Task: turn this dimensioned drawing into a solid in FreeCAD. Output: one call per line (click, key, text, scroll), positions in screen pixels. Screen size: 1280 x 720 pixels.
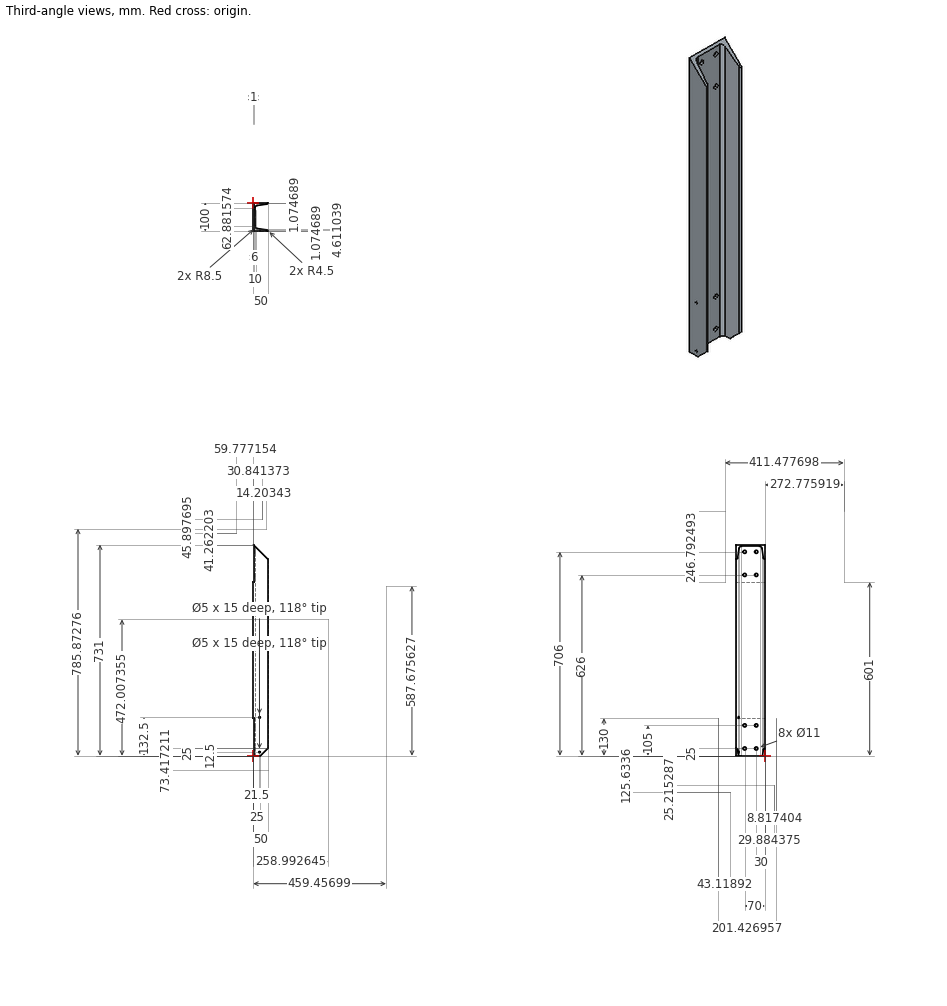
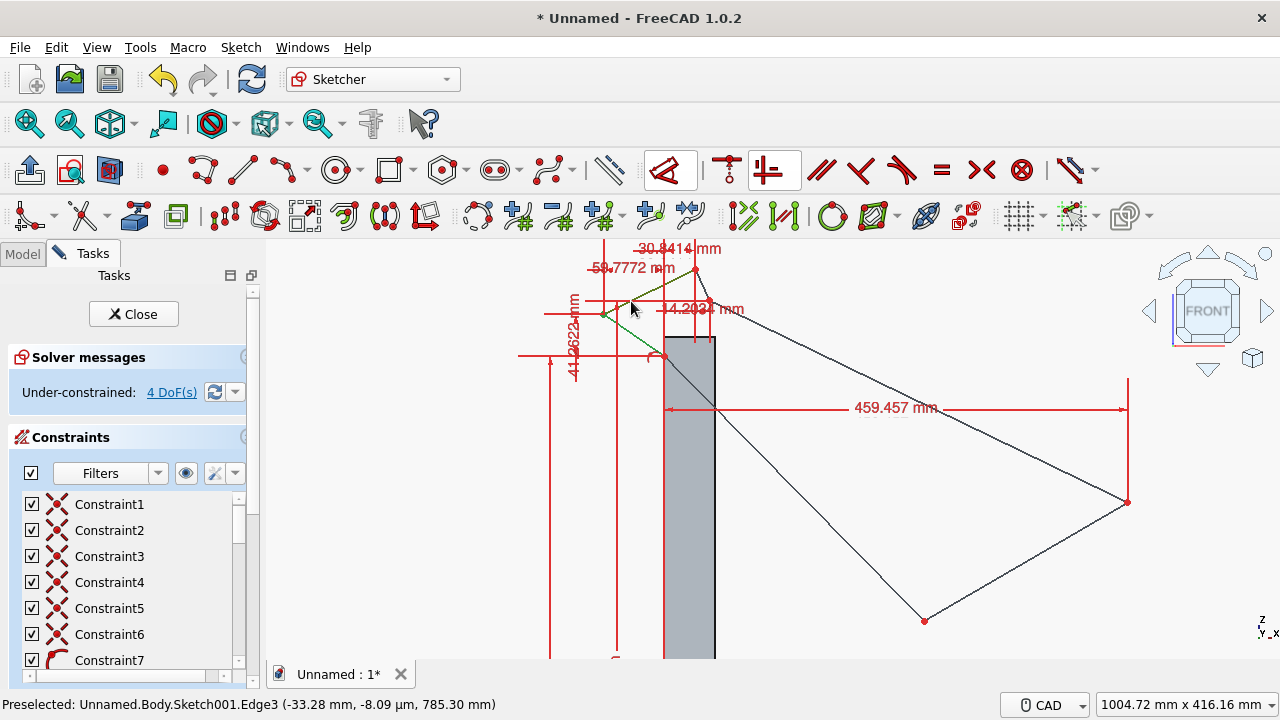
key(i)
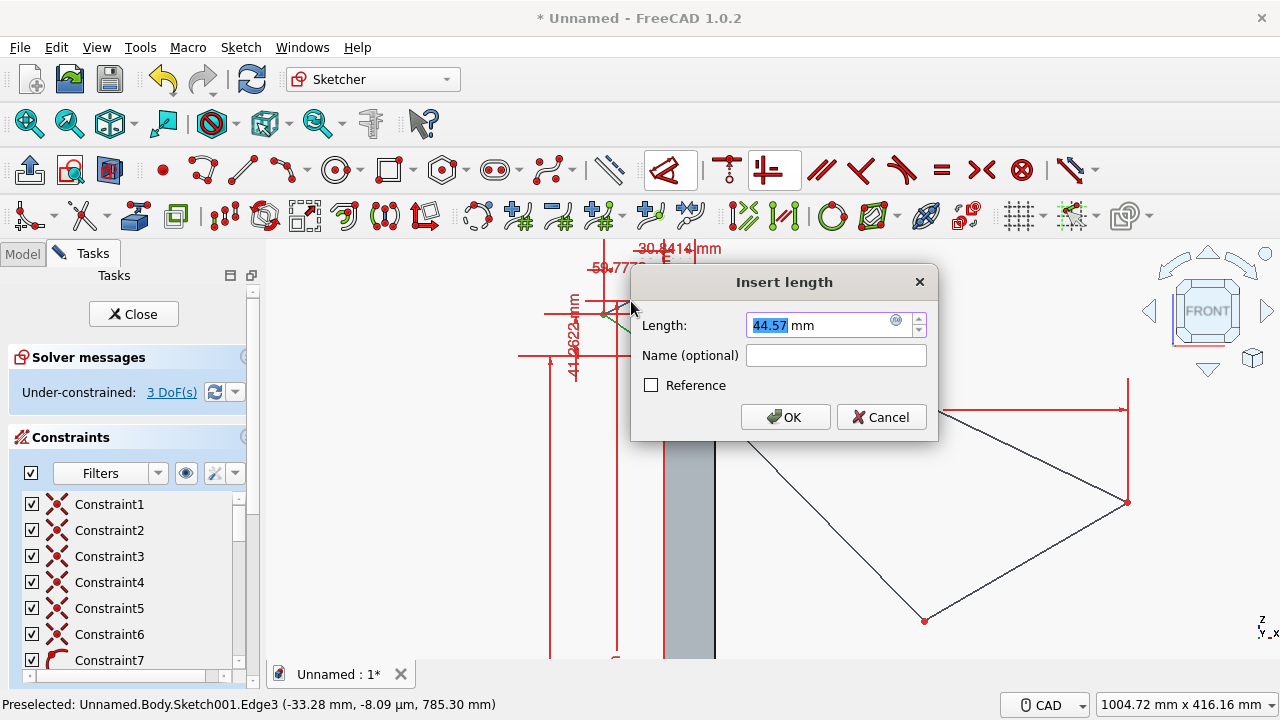
text(45.897695)
key(Return)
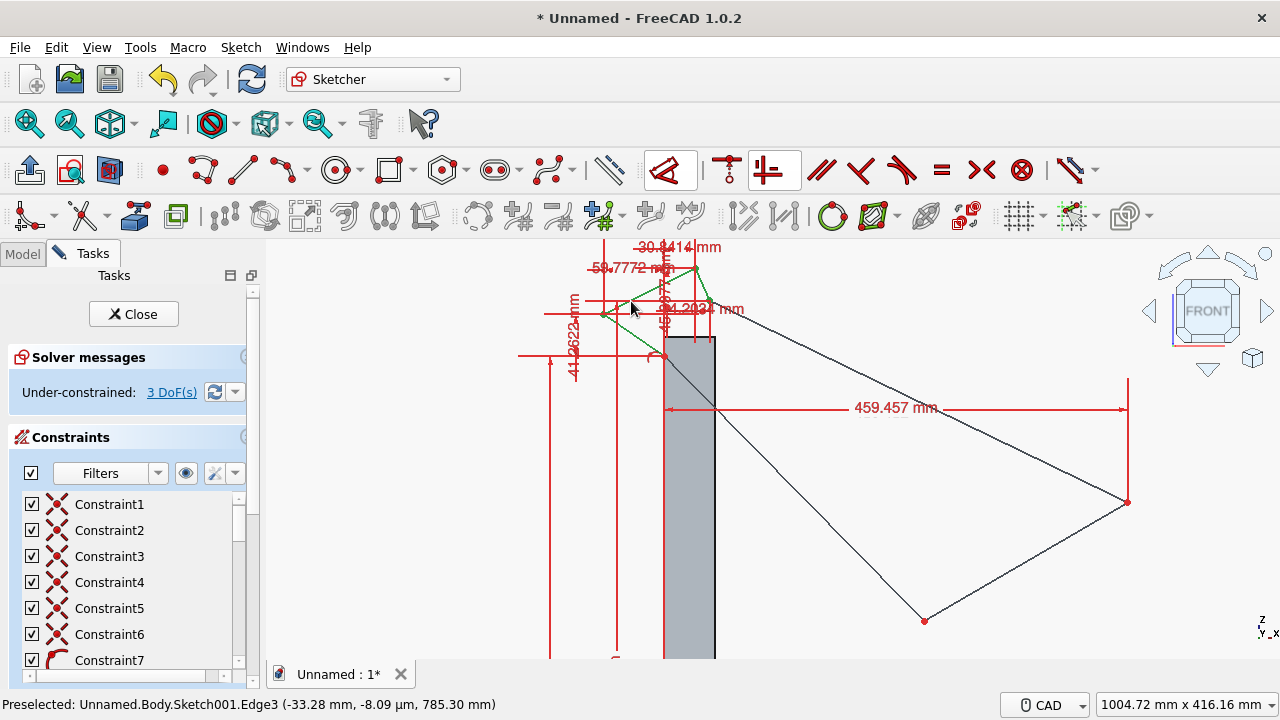
click(924, 621)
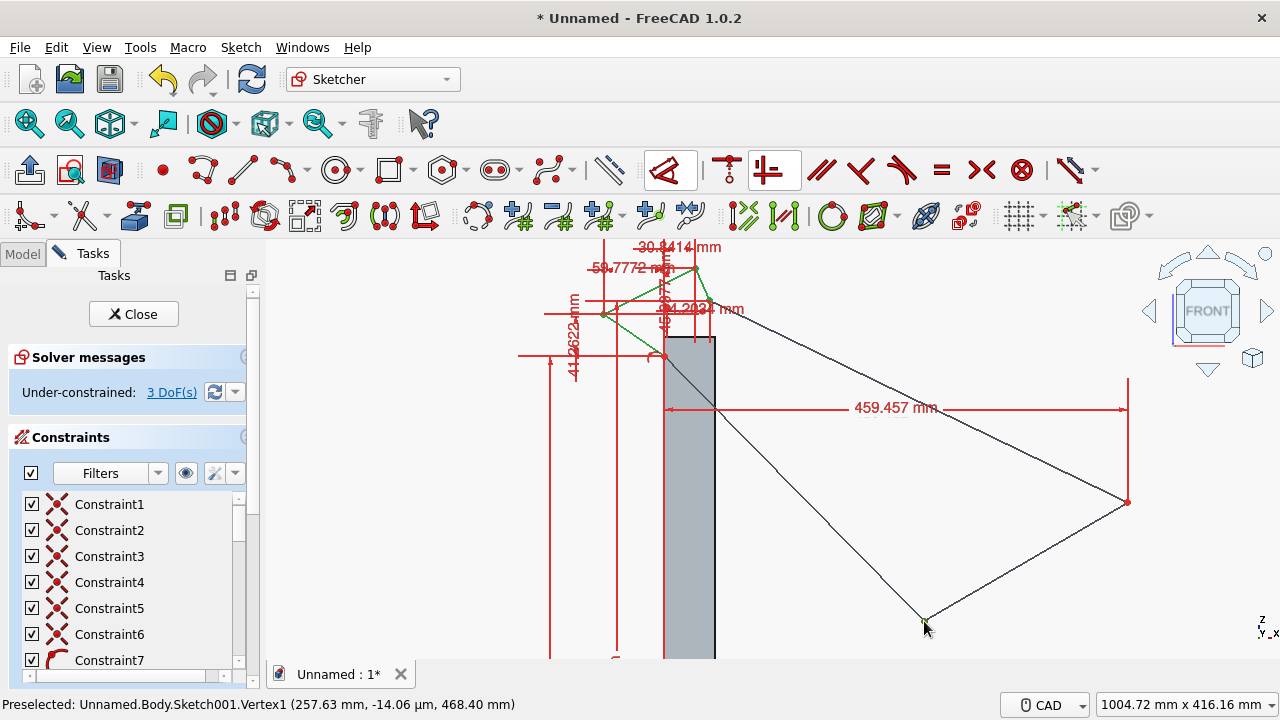
key(l)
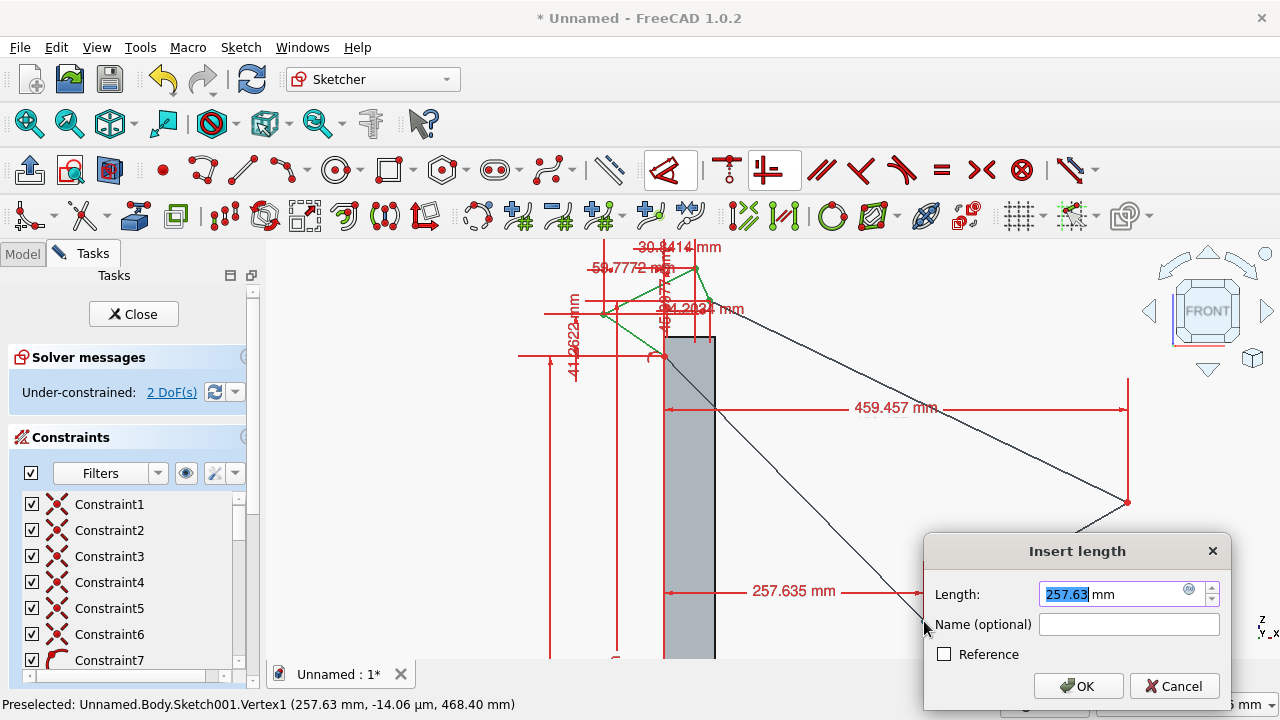
text(258.992645)
key(Return)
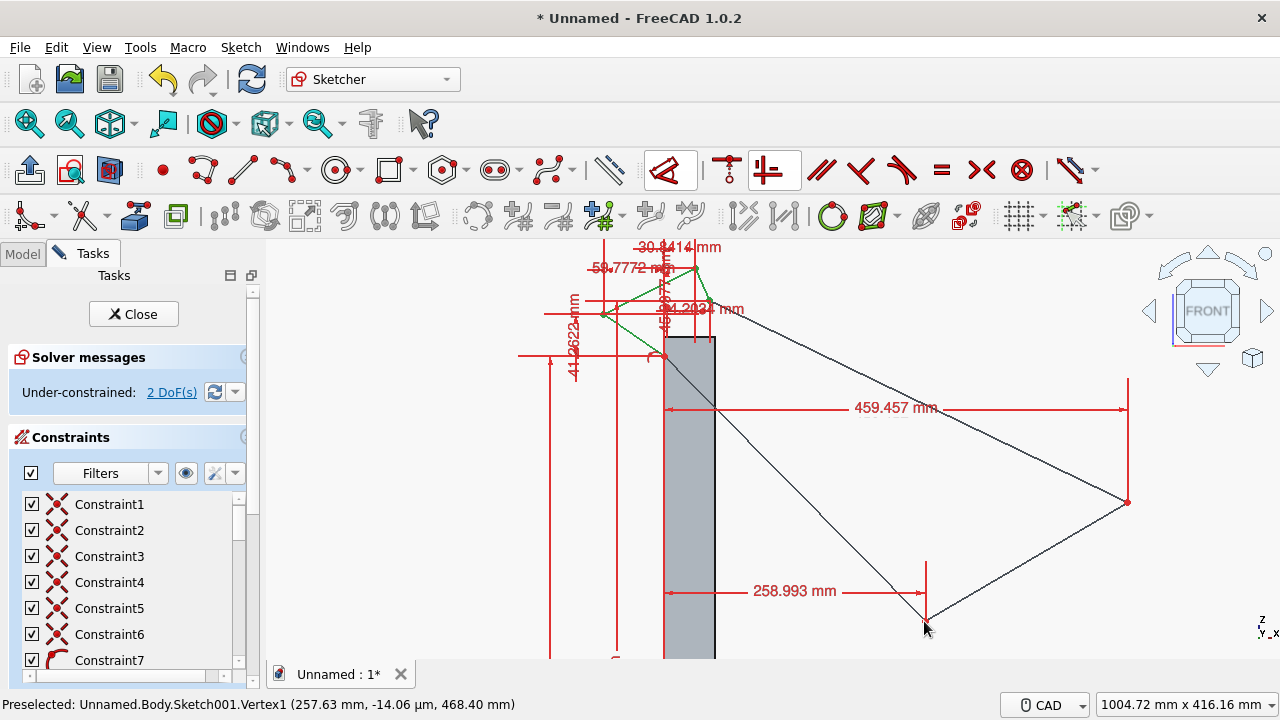
click(926, 621)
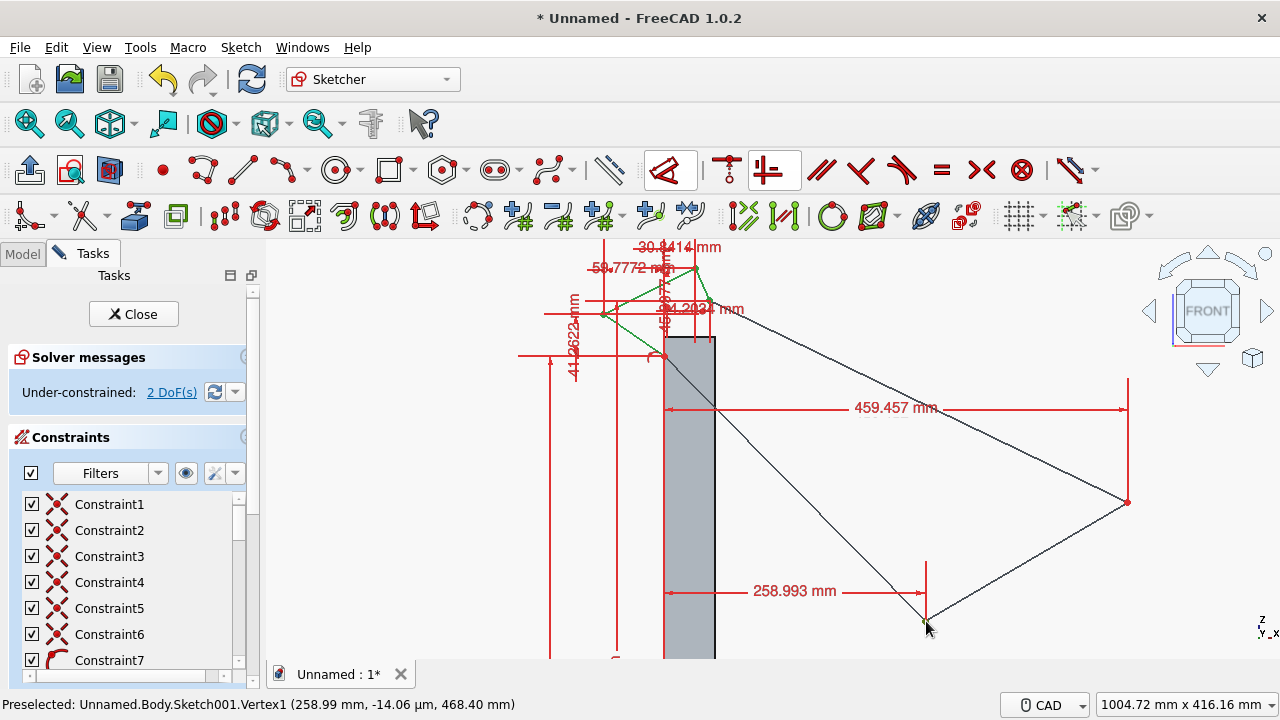
click(692, 170)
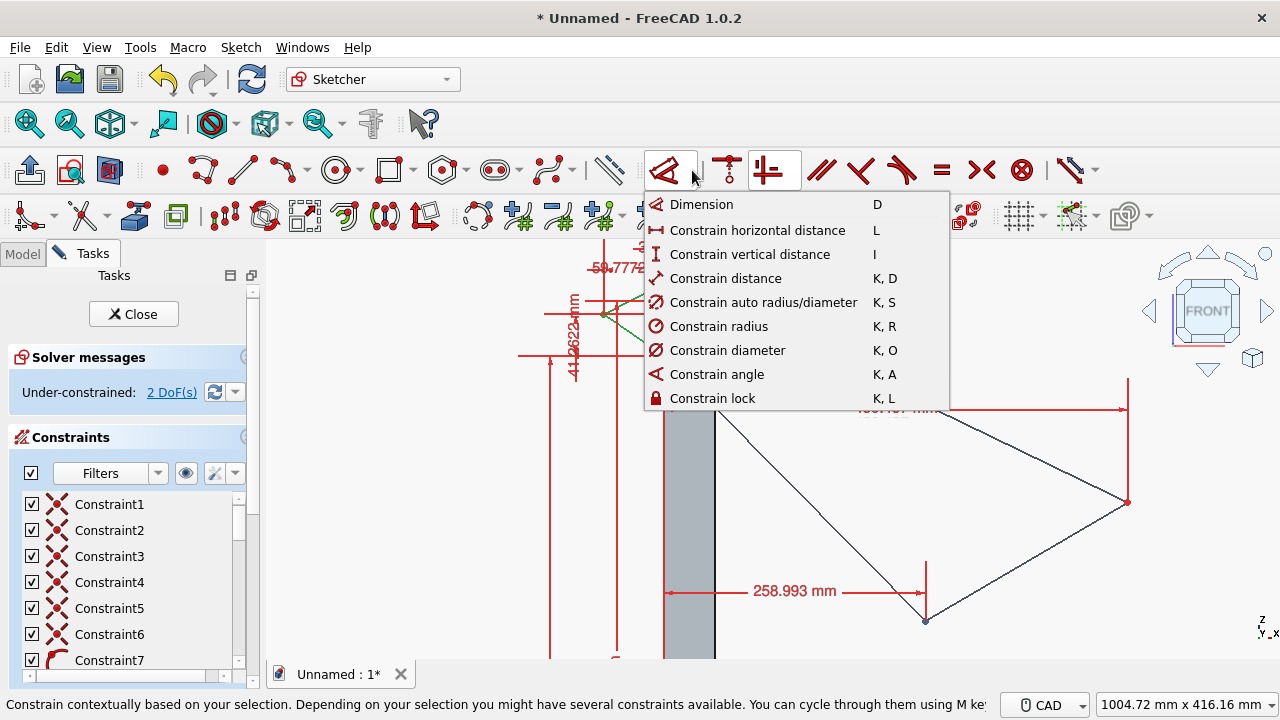
click(797, 254)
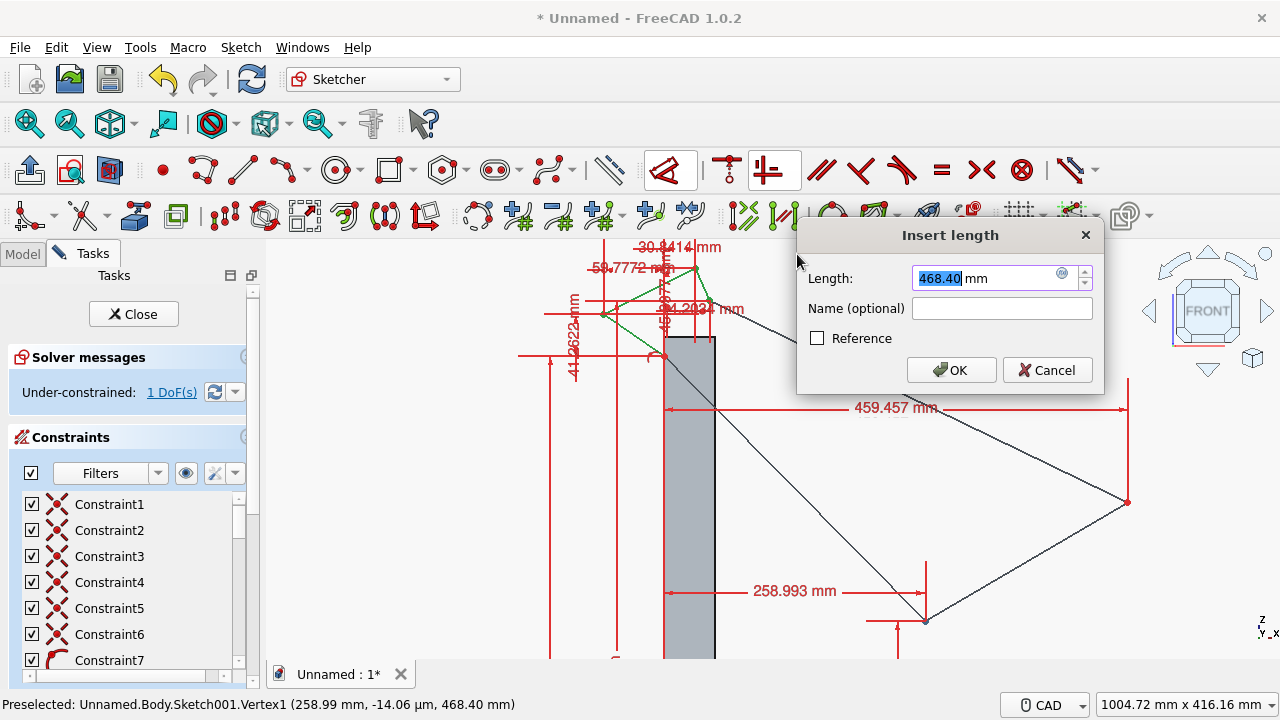
text(472.007355)
key(Return)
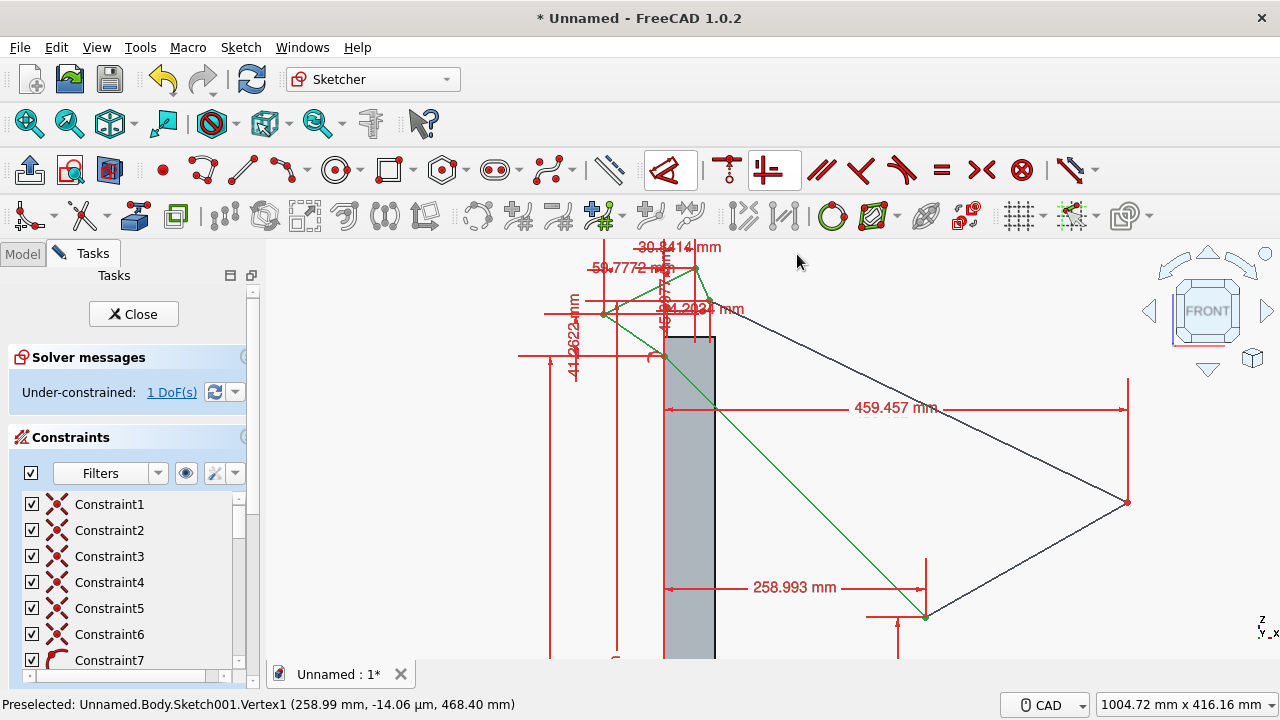
scroll(635, 339, down, 6)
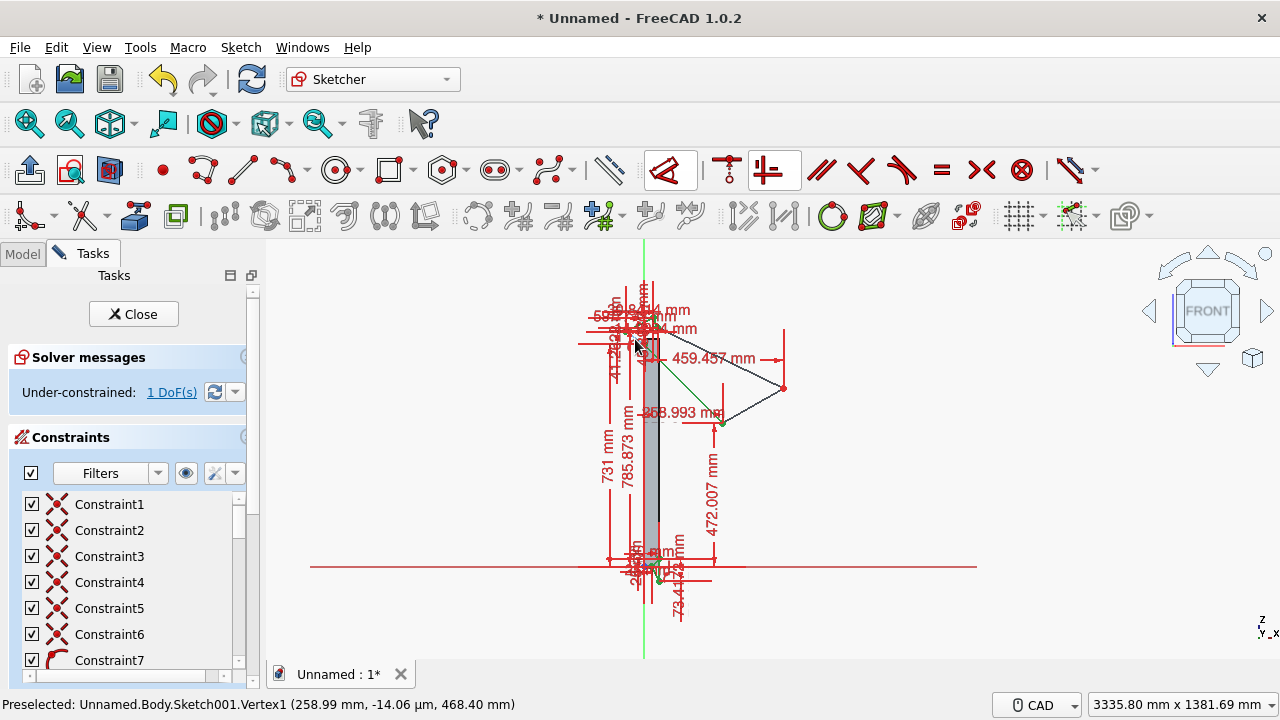
click(784, 388)